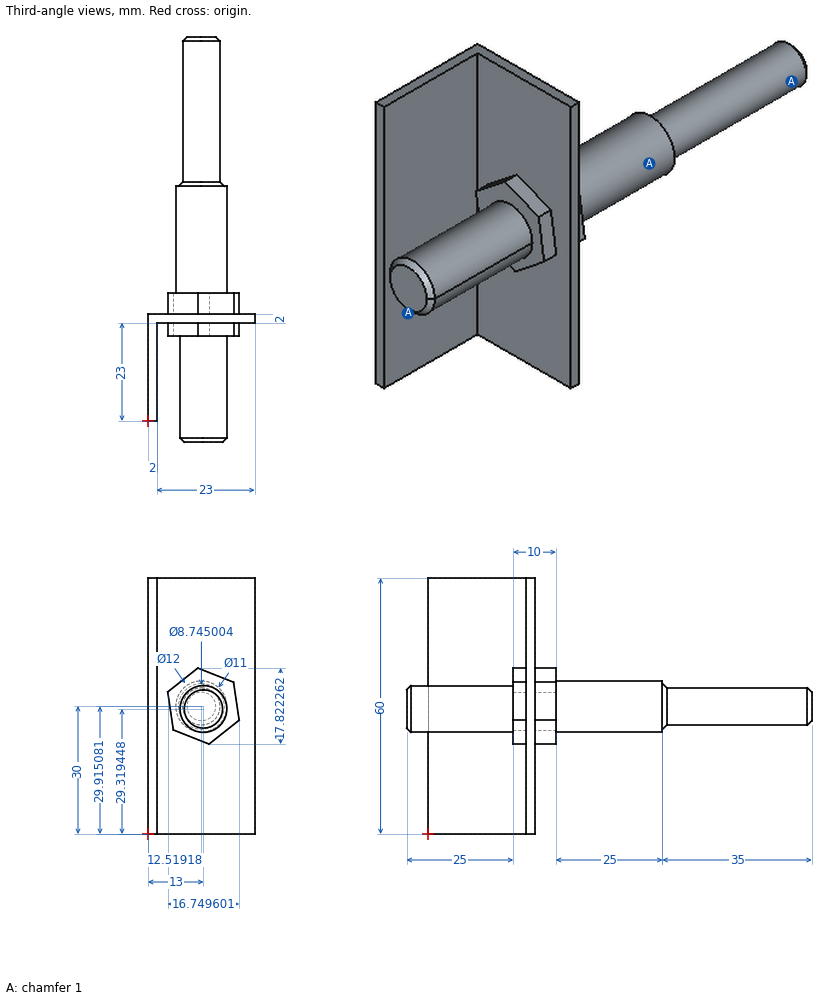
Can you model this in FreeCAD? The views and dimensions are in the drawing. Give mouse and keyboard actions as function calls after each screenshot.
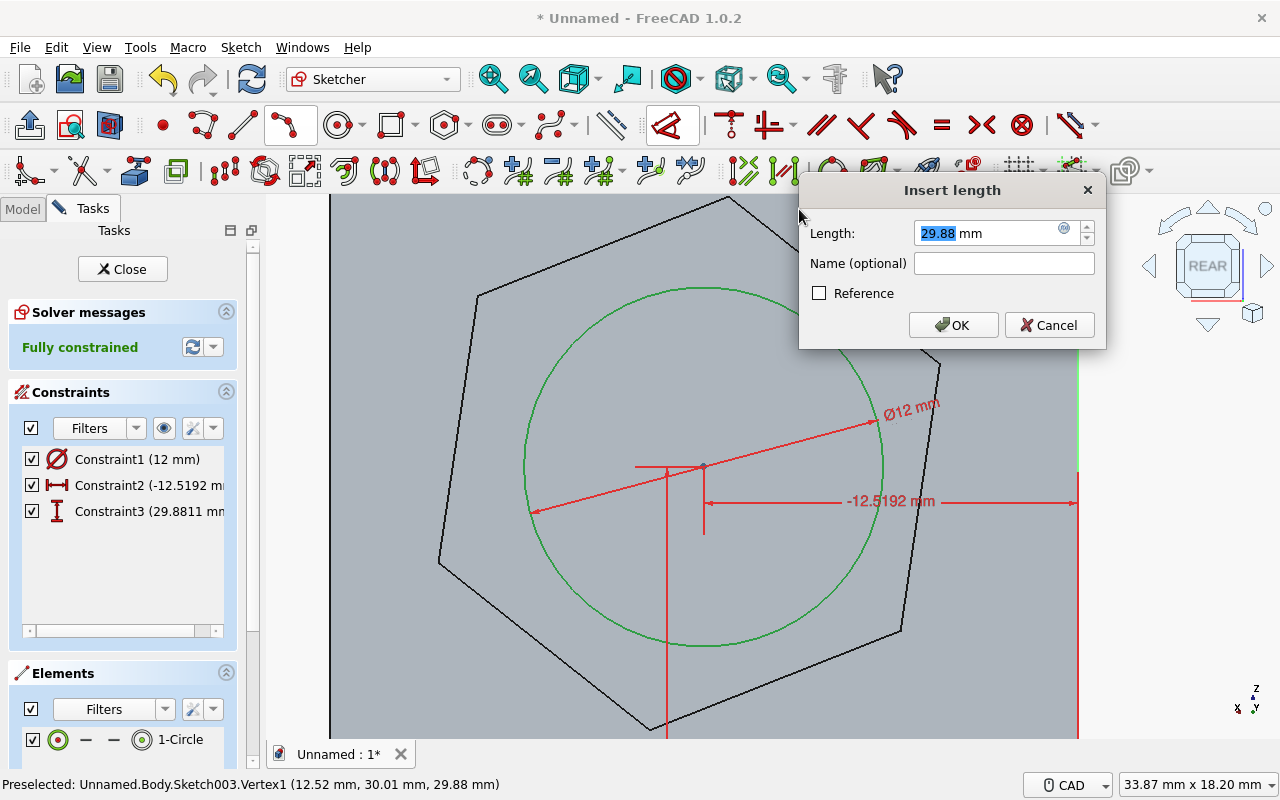
text(29.915081)
key(Return)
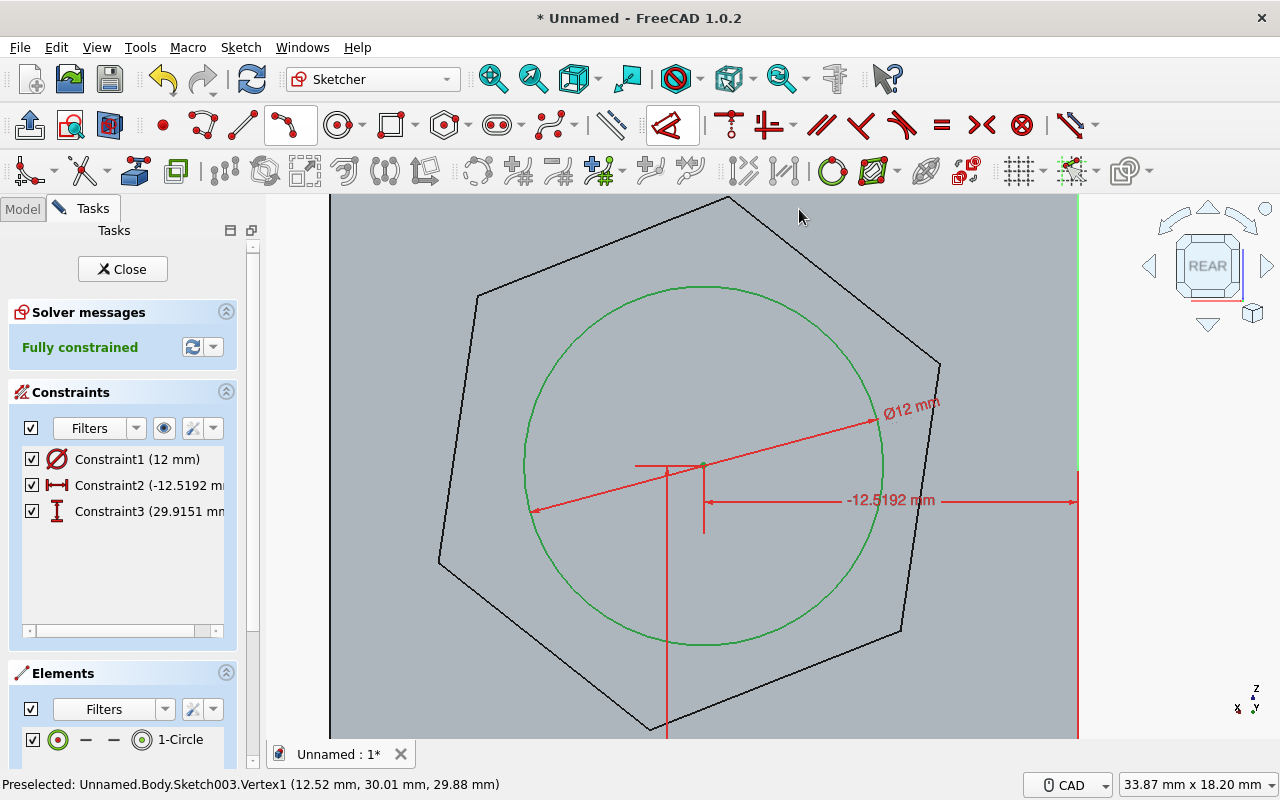
click(123, 269)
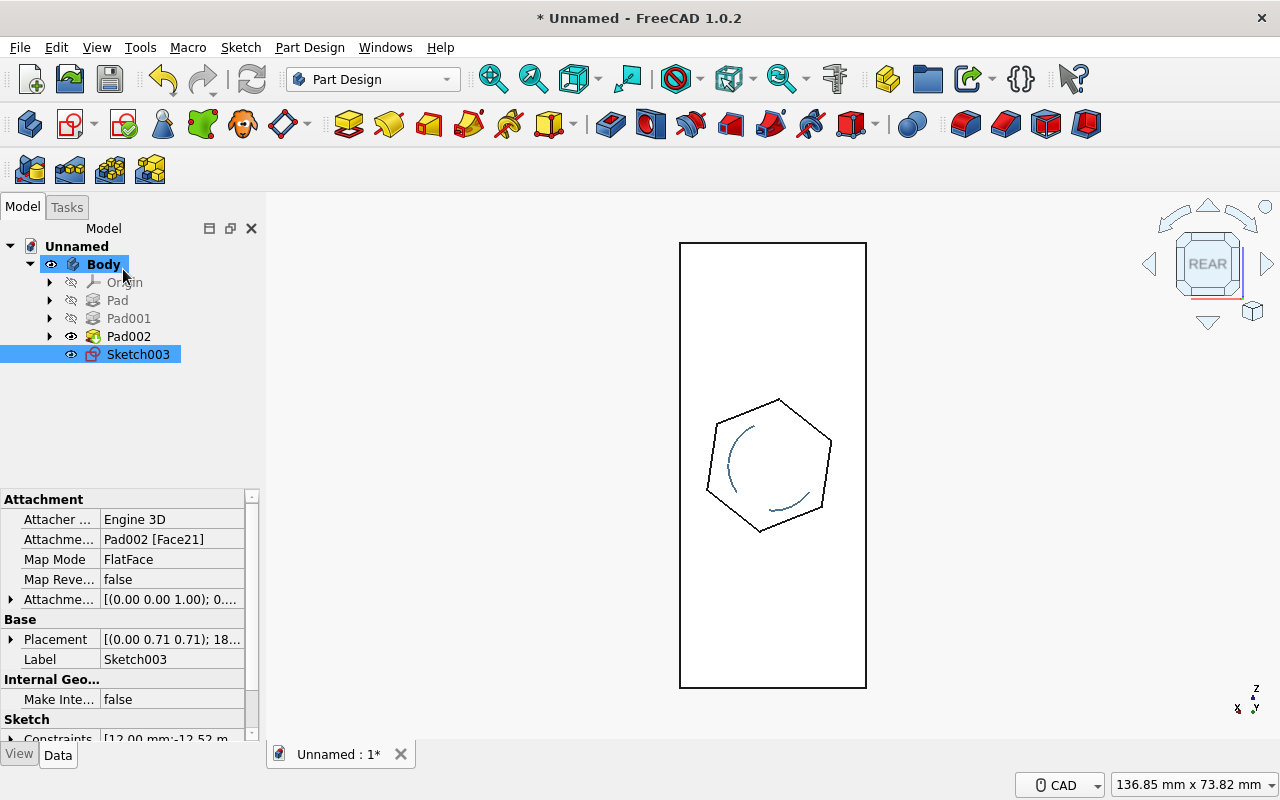
click(350, 124)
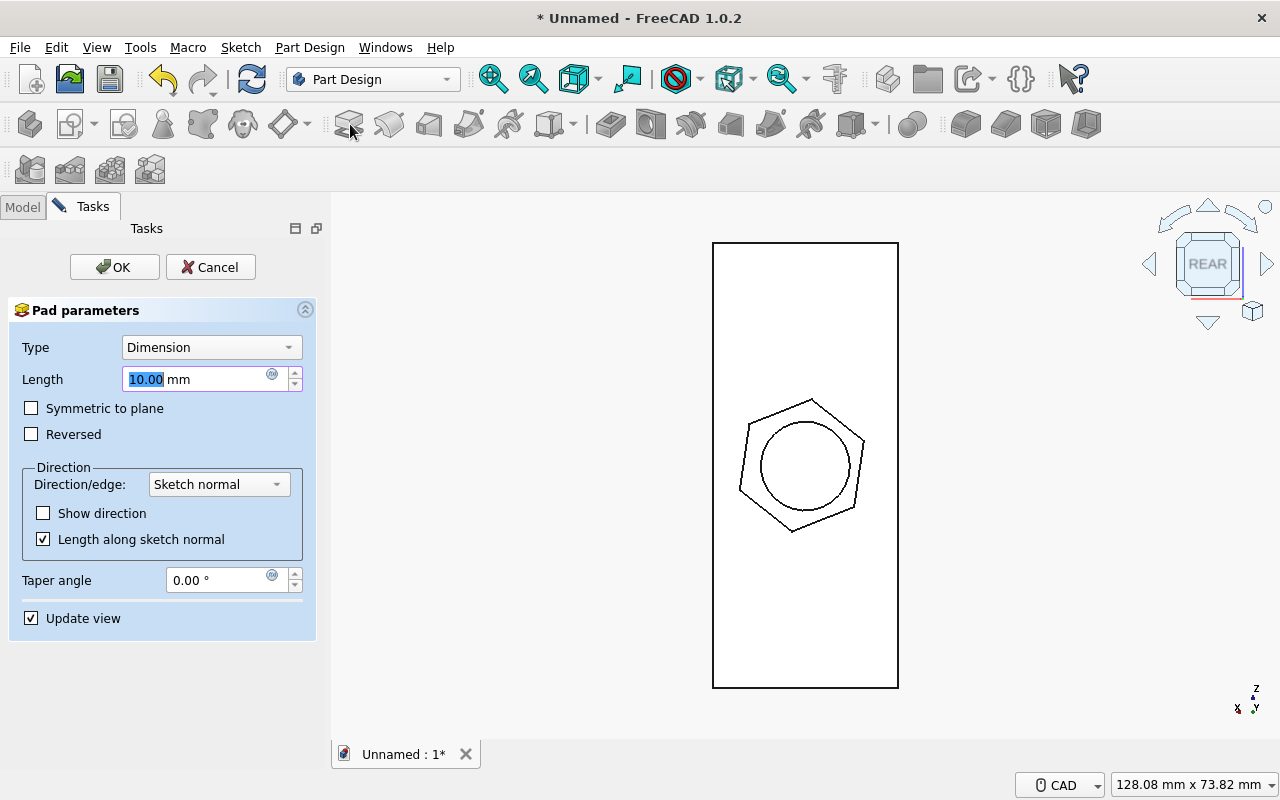
text(25)
key(Tab)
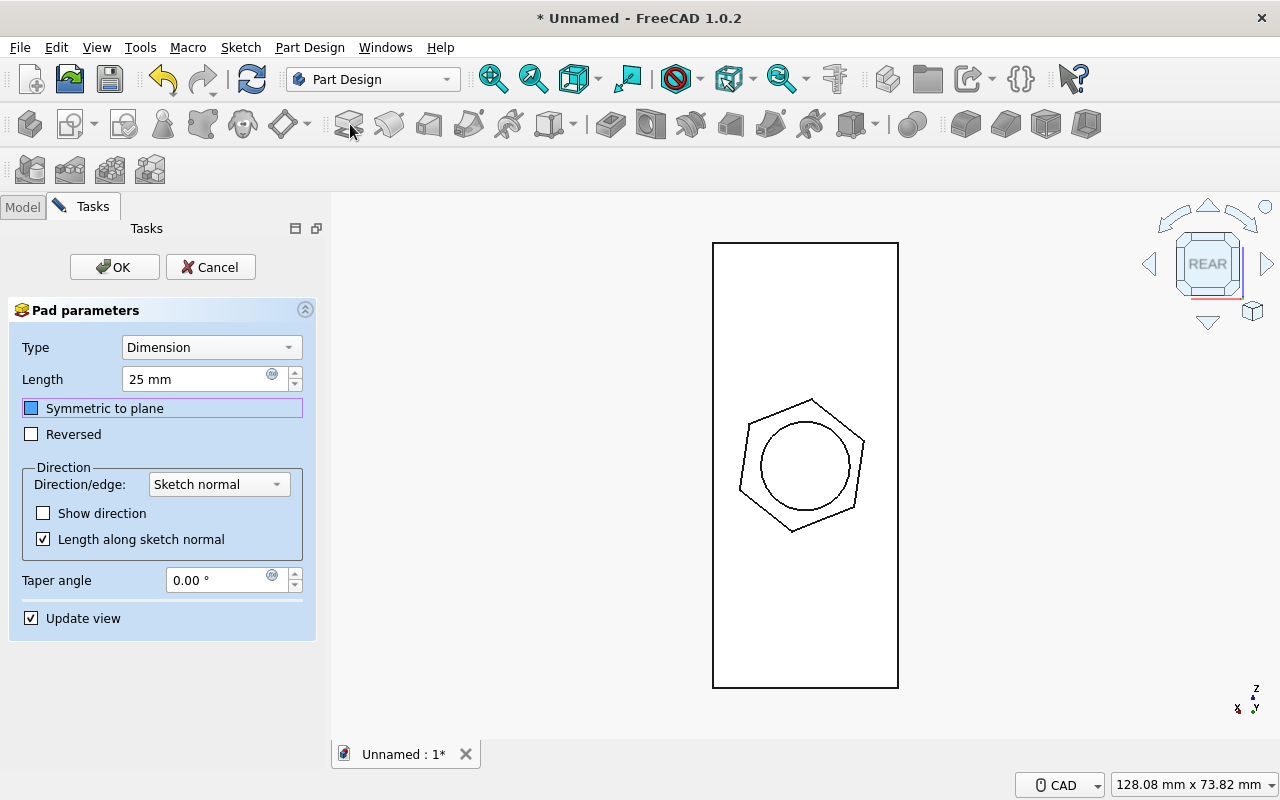
click(115, 267)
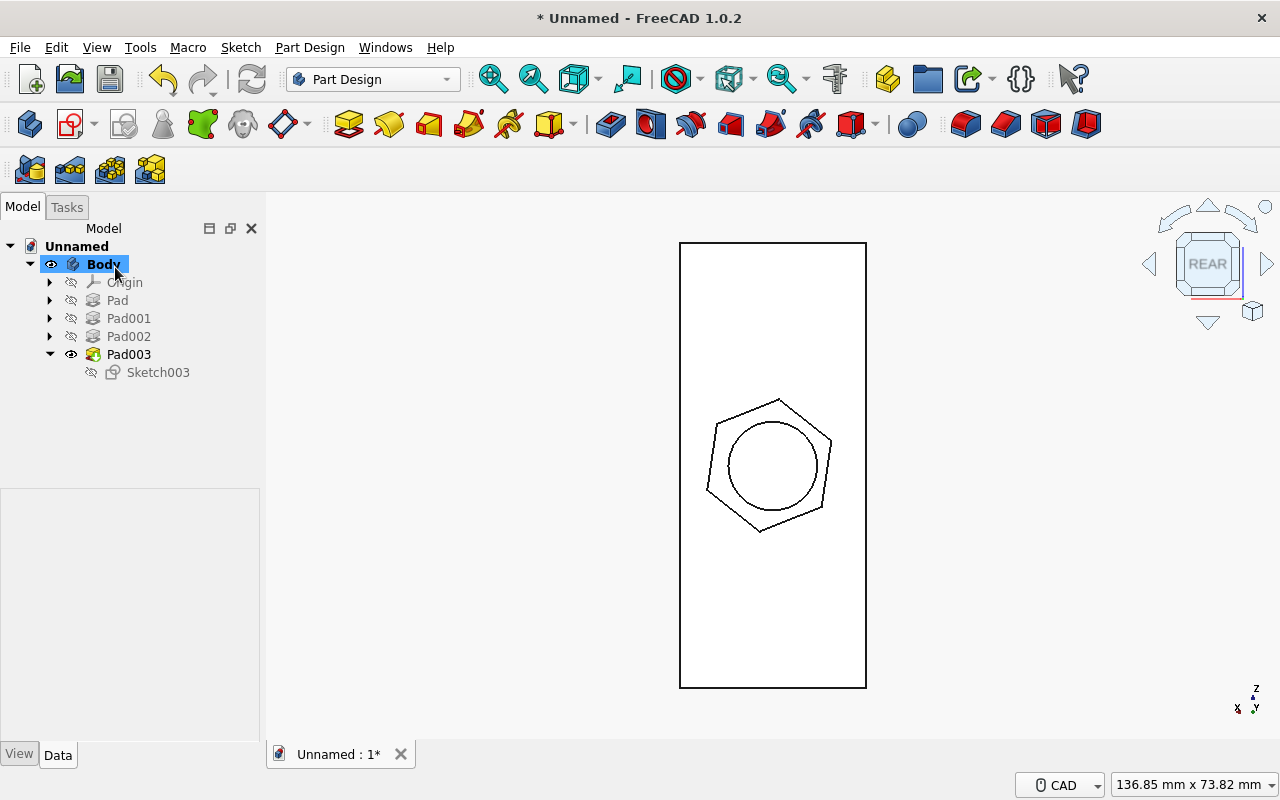
click(773, 465)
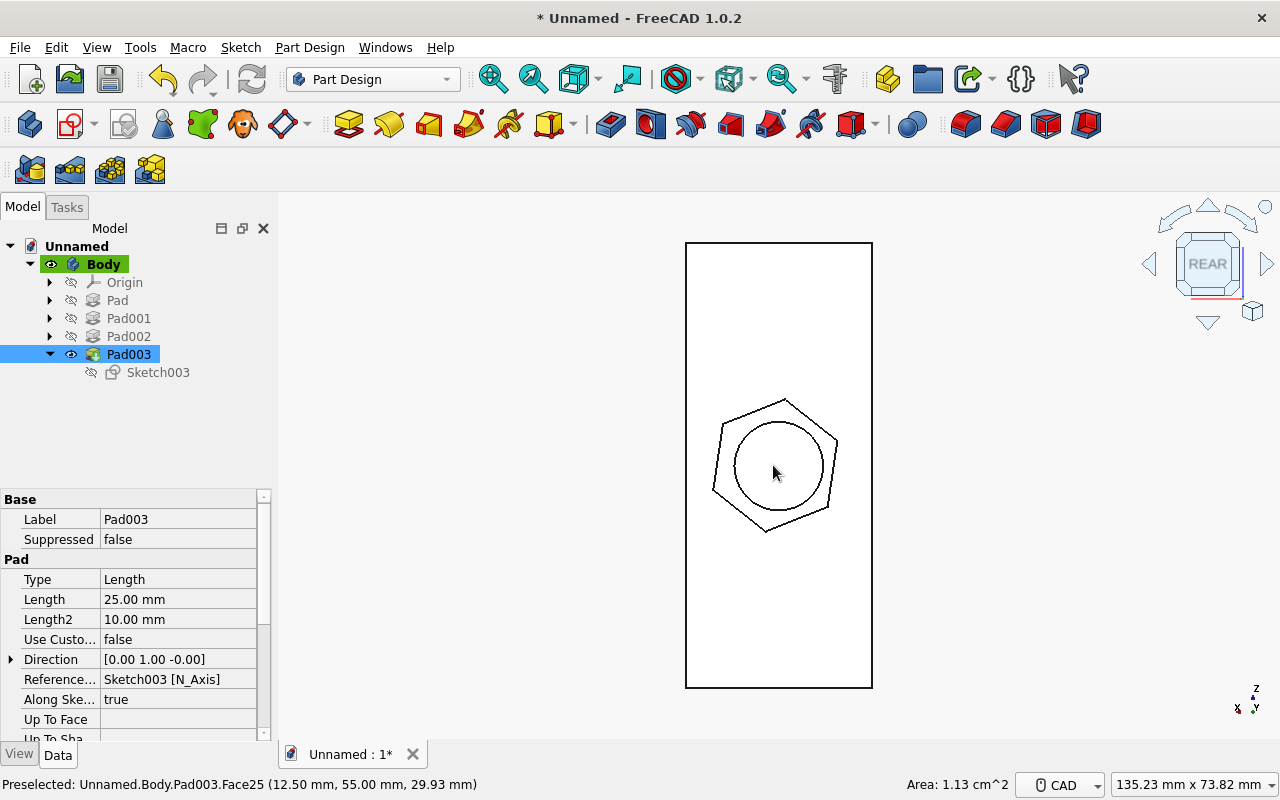
click(70, 124)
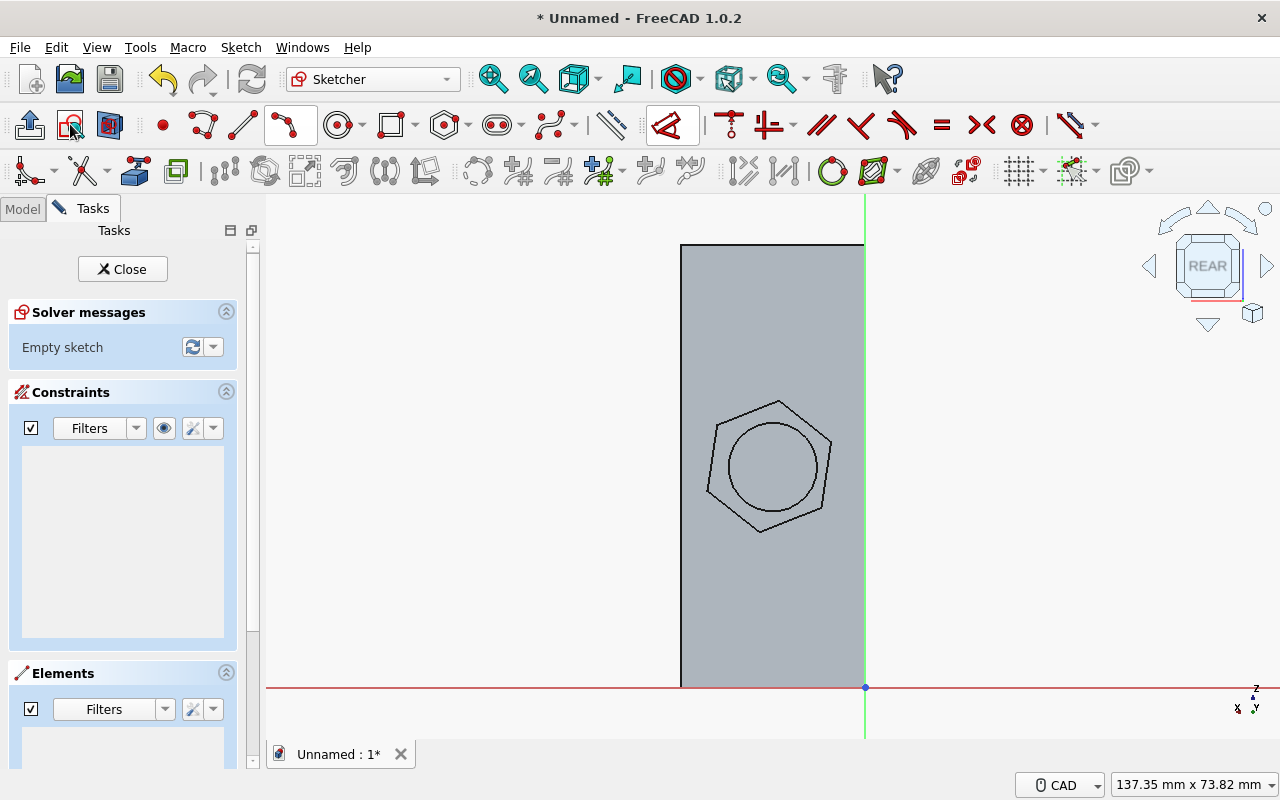
scroll(790, 467, up, 8)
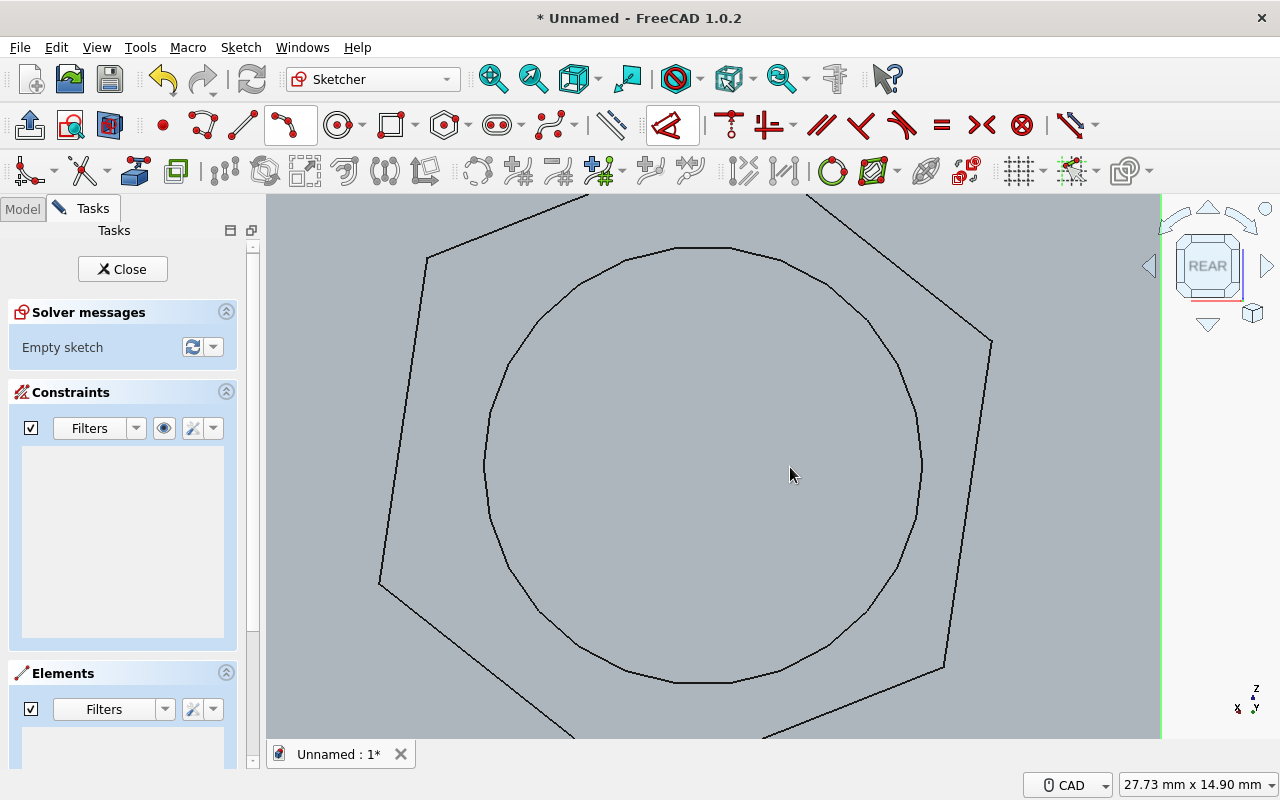
key(g)
key(c)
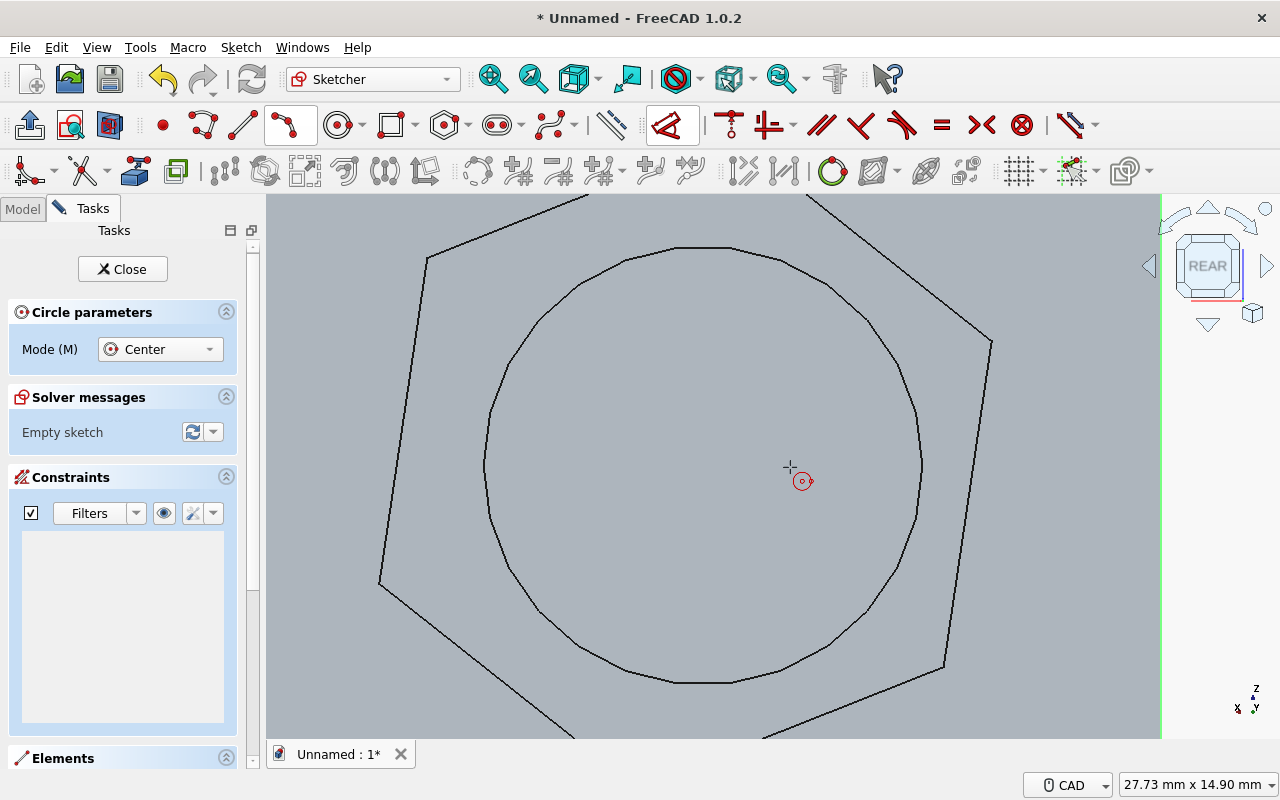
click(703, 466)
click(816, 353)
key(Escape)